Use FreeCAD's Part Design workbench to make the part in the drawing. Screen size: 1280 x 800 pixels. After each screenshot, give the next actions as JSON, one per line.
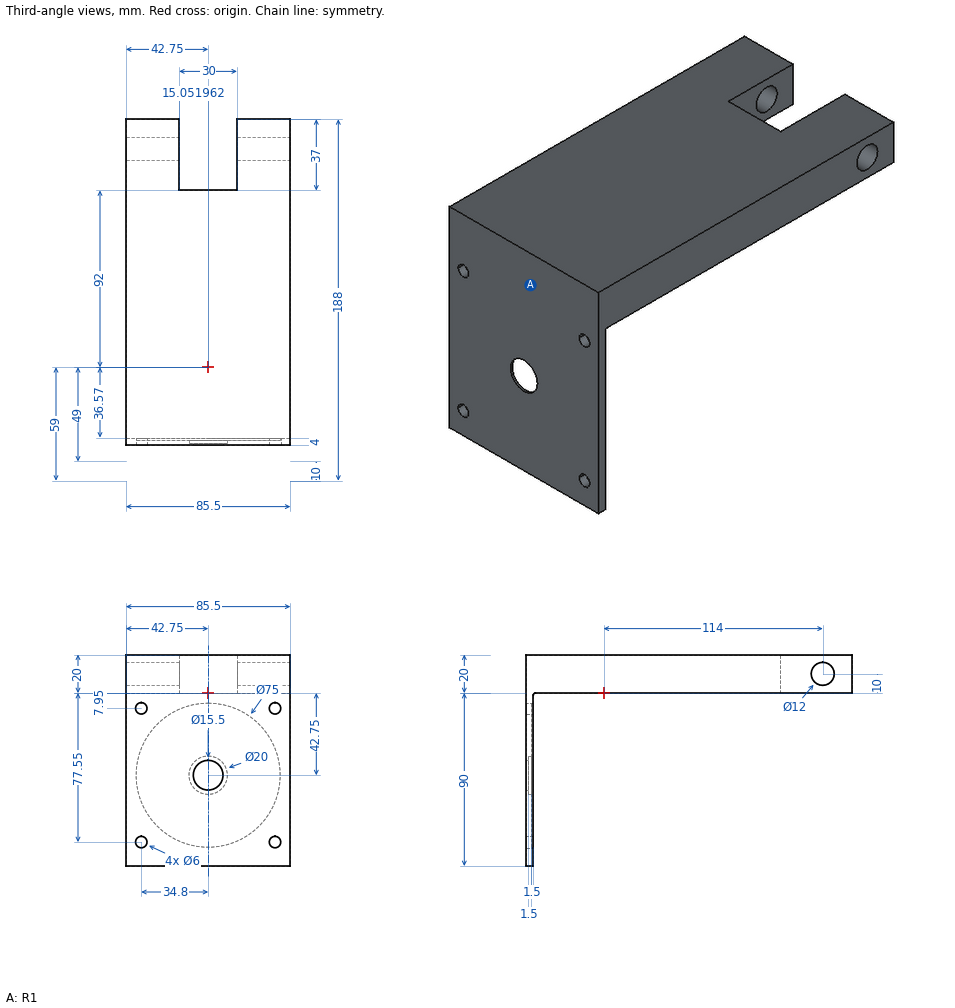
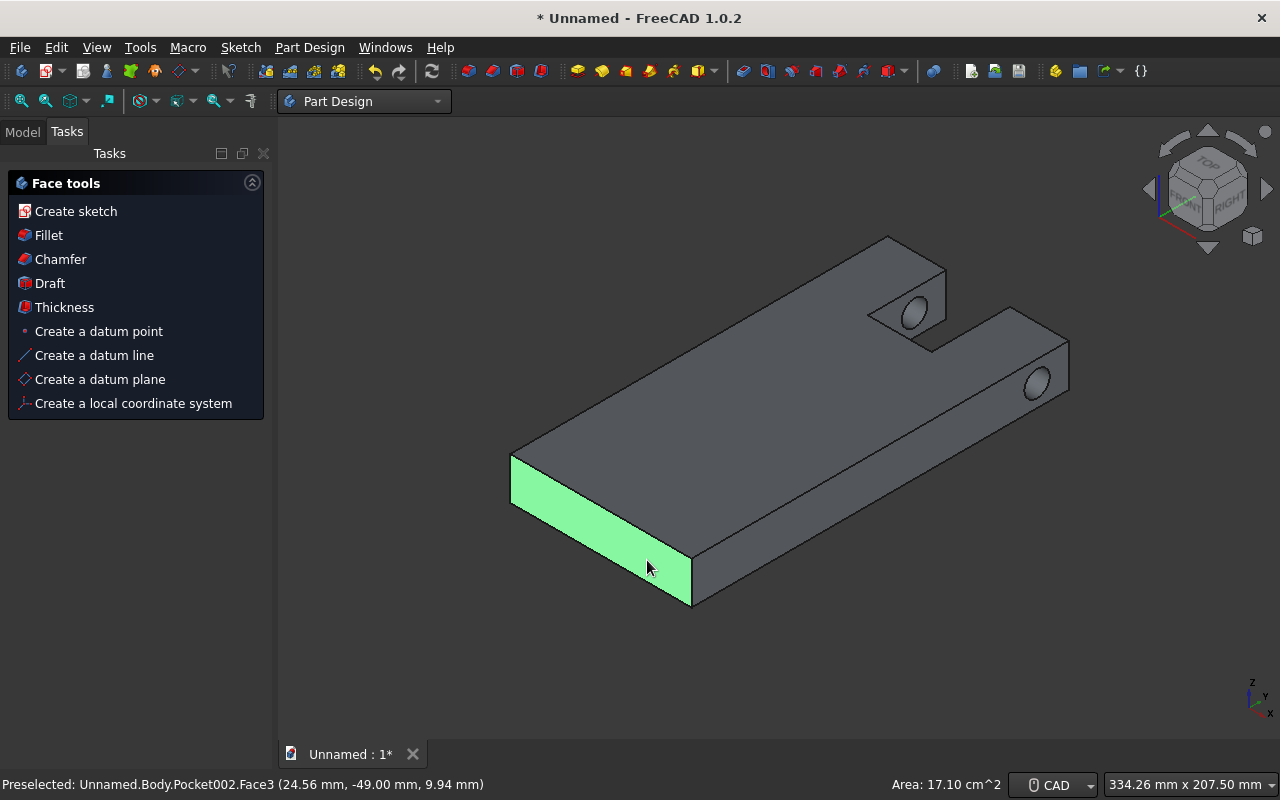
{"action": "left_click", "coordinate": [46, 72]}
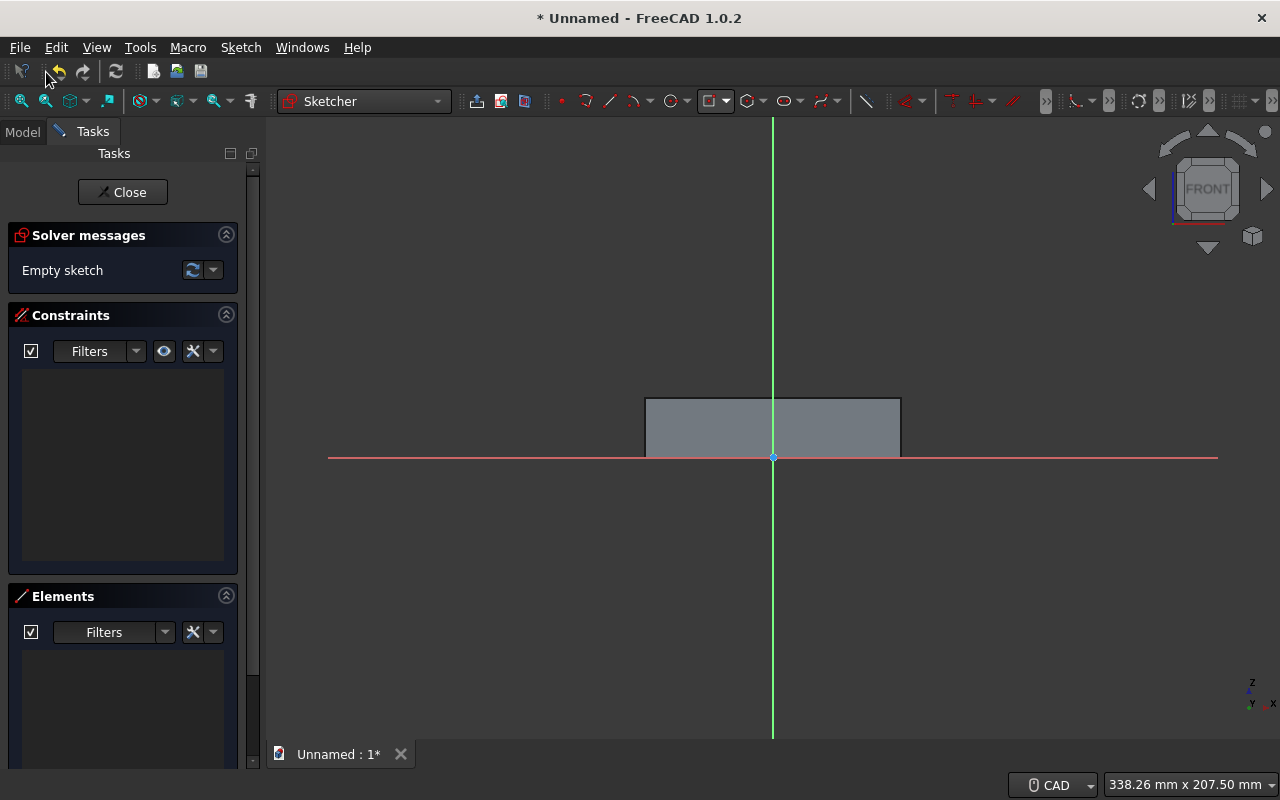
{"action": "scroll", "coordinate": [829, 428], "scroll_direction": "up", "scroll_amount": 4}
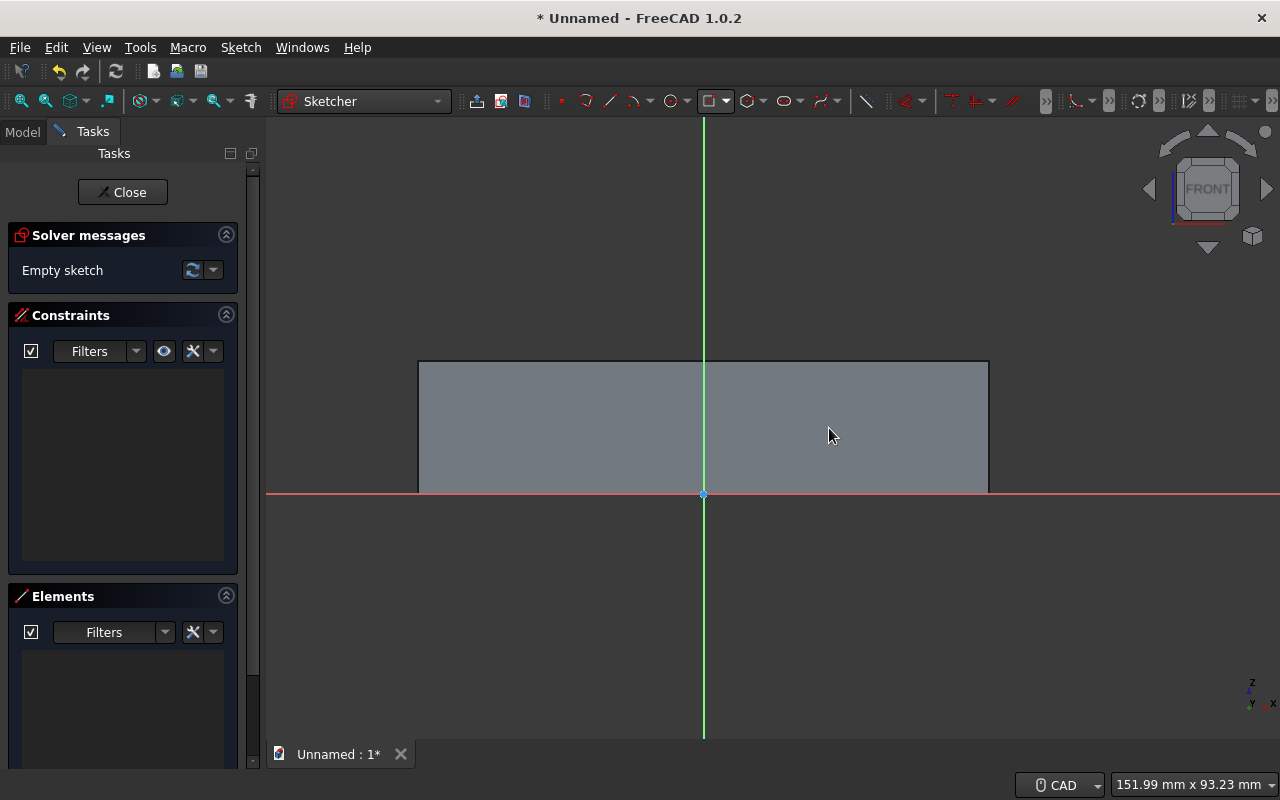
{"action": "left_click", "coordinate": [728, 102]}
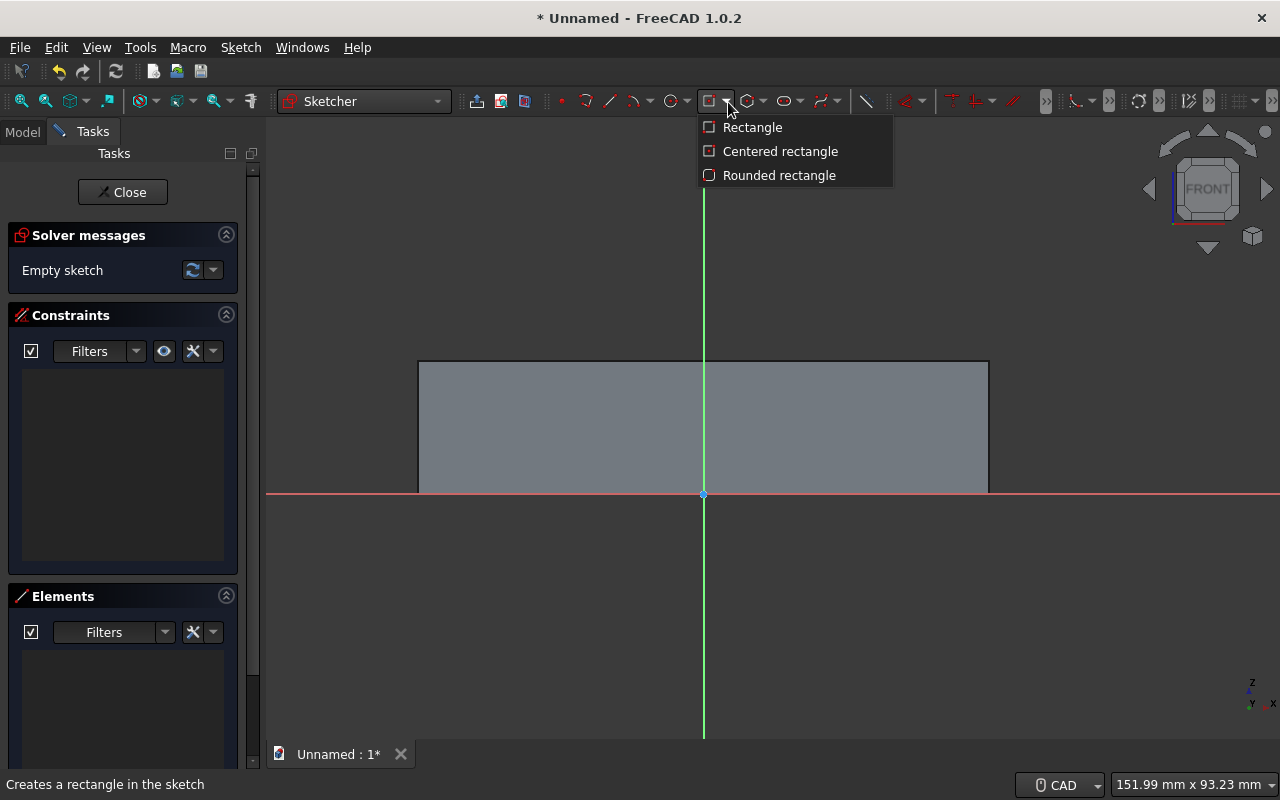
{"action": "left_click", "coordinate": [796, 127]}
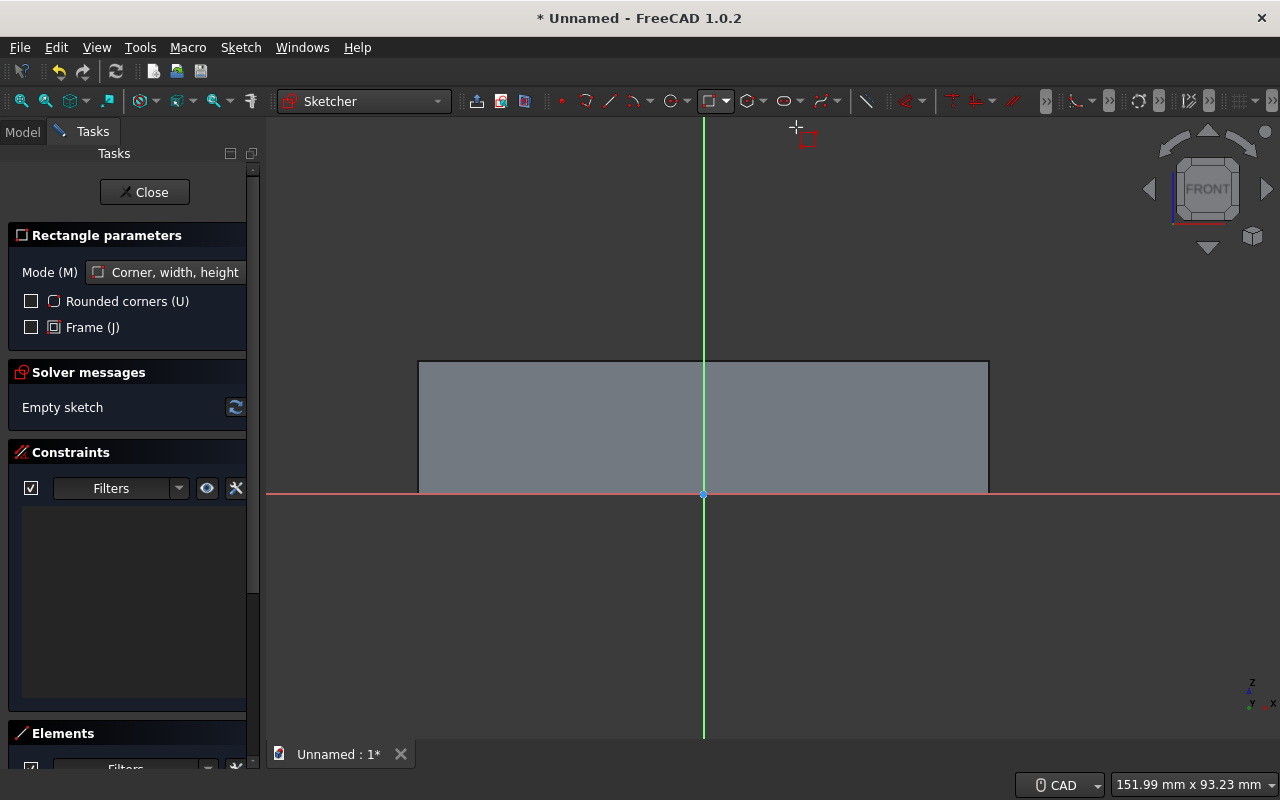
{"action": "left_click", "coordinate": [418, 361]}
{"action": "left_click", "coordinate": [989, 494]}
{"action": "key", "text": "Escape"}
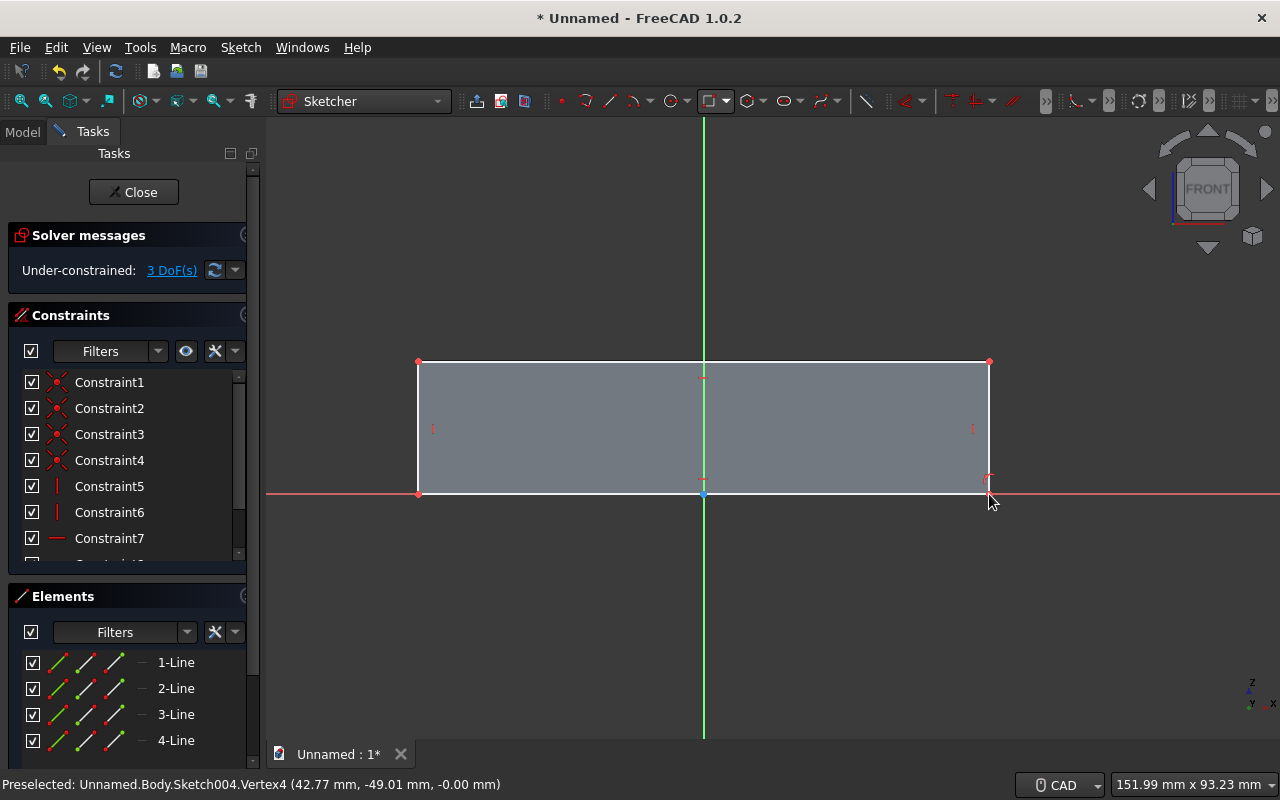
{"action": "key", "text": "d"}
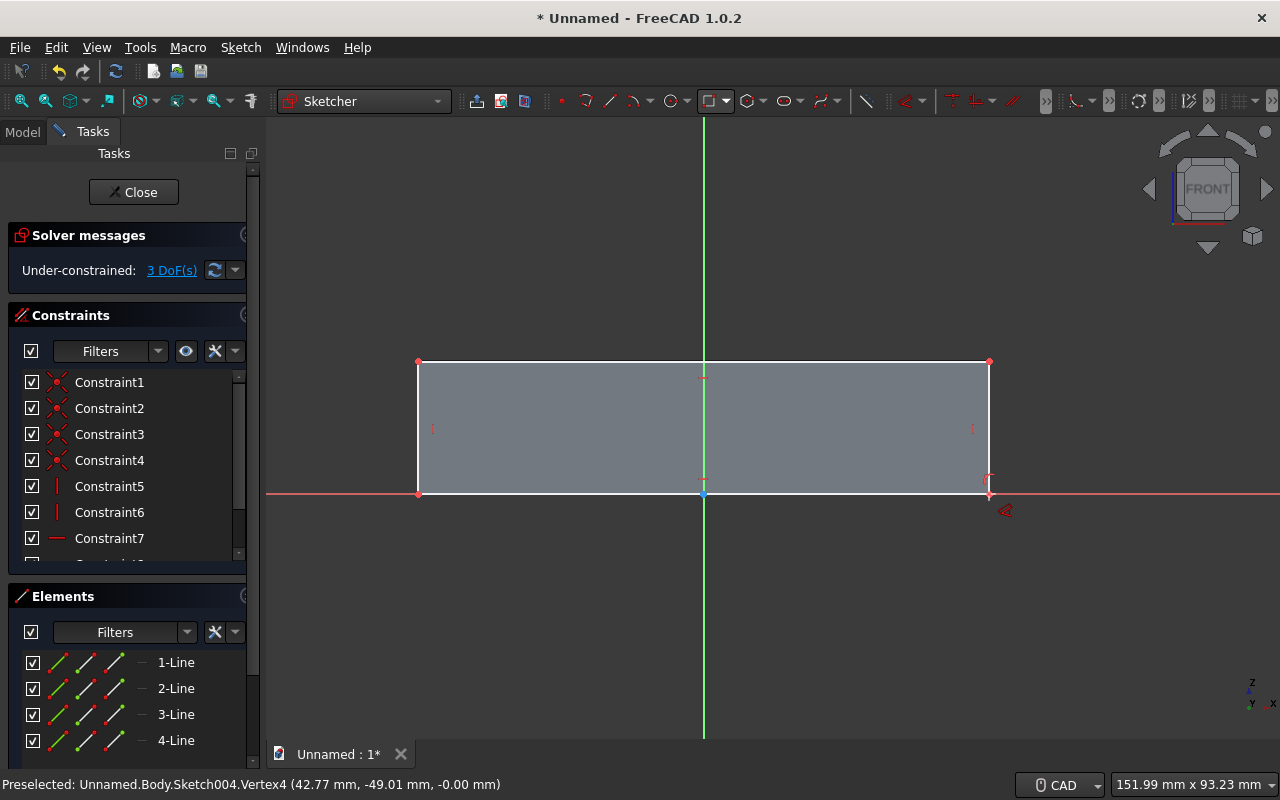
{"action": "left_click", "coordinate": [418, 402]}
{"action": "left_click", "coordinate": [384, 428]}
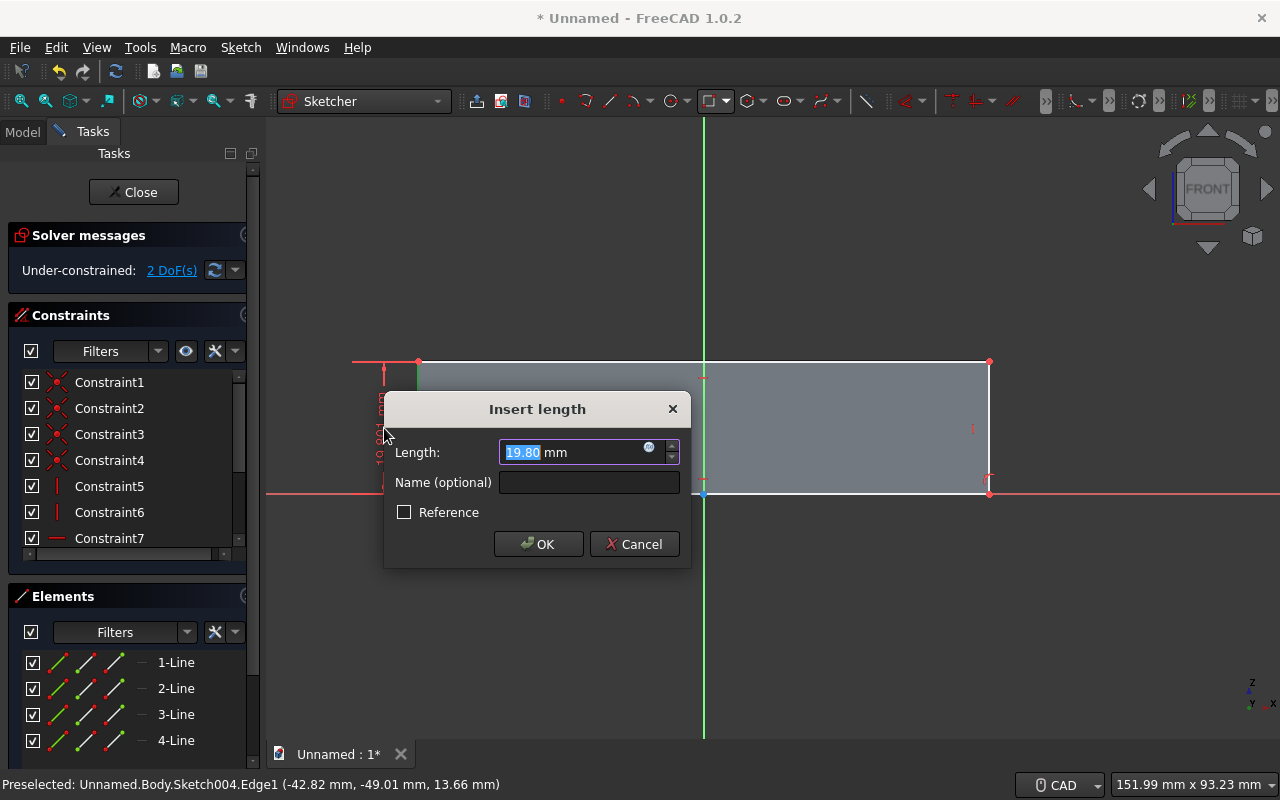
{"action": "type", "text": "20"}
{"action": "key", "text": "Return"}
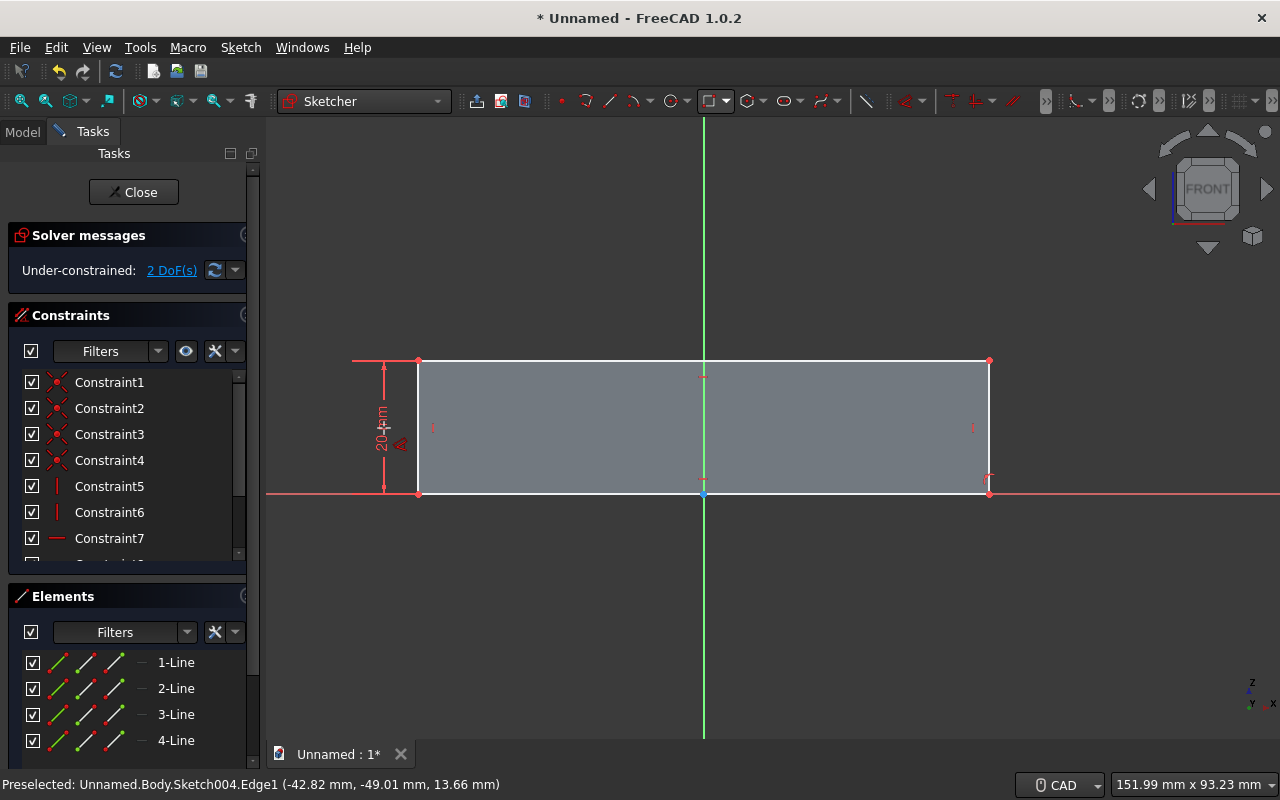
{"action": "left_click", "coordinate": [589, 494]}
{"action": "left_click", "coordinate": [572, 528]}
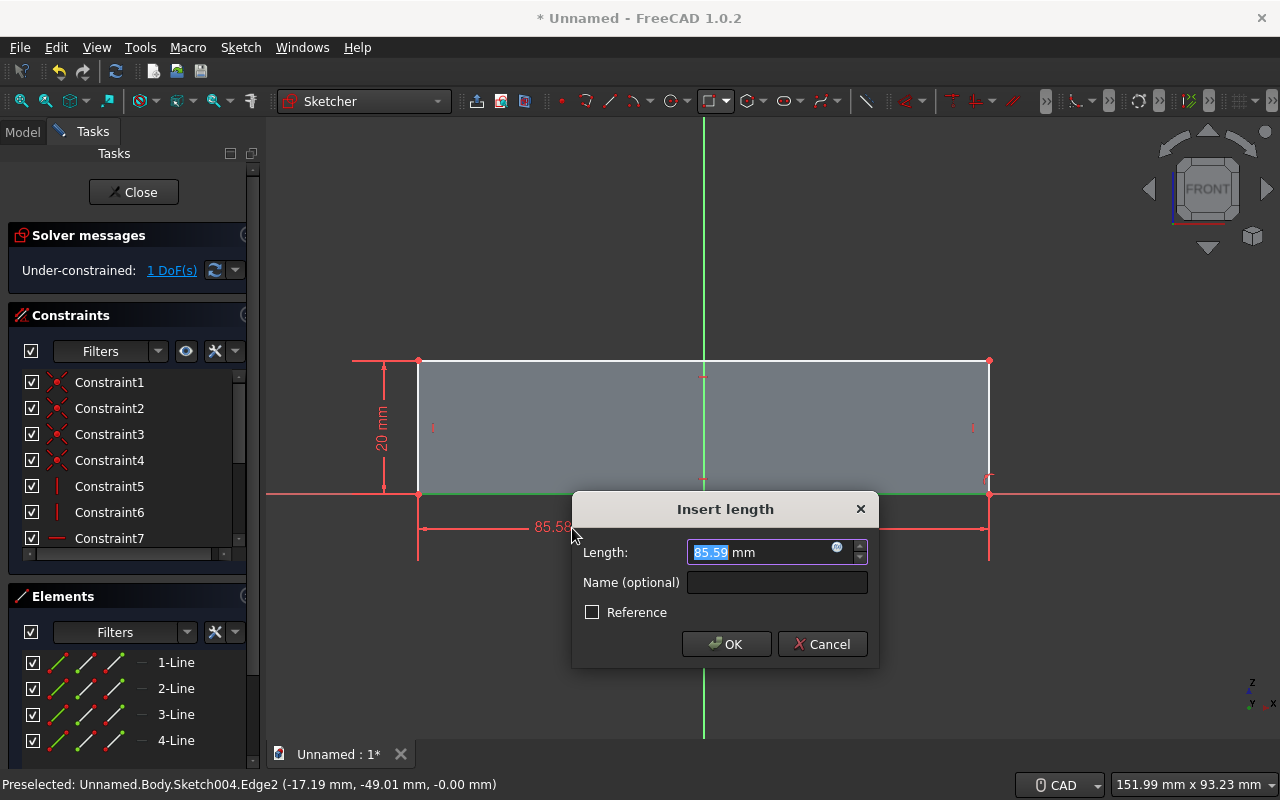
{"action": "type", "text": "85.5"}
{"action": "key", "text": "Return"}